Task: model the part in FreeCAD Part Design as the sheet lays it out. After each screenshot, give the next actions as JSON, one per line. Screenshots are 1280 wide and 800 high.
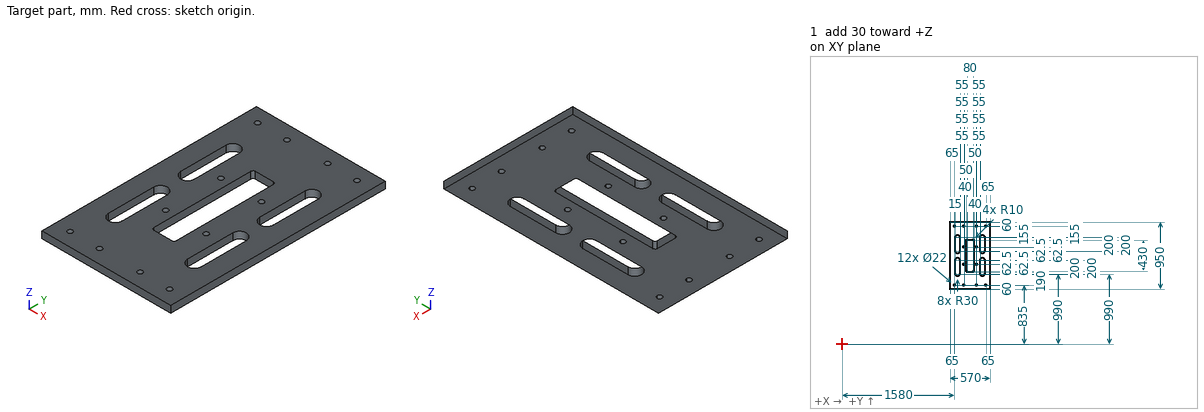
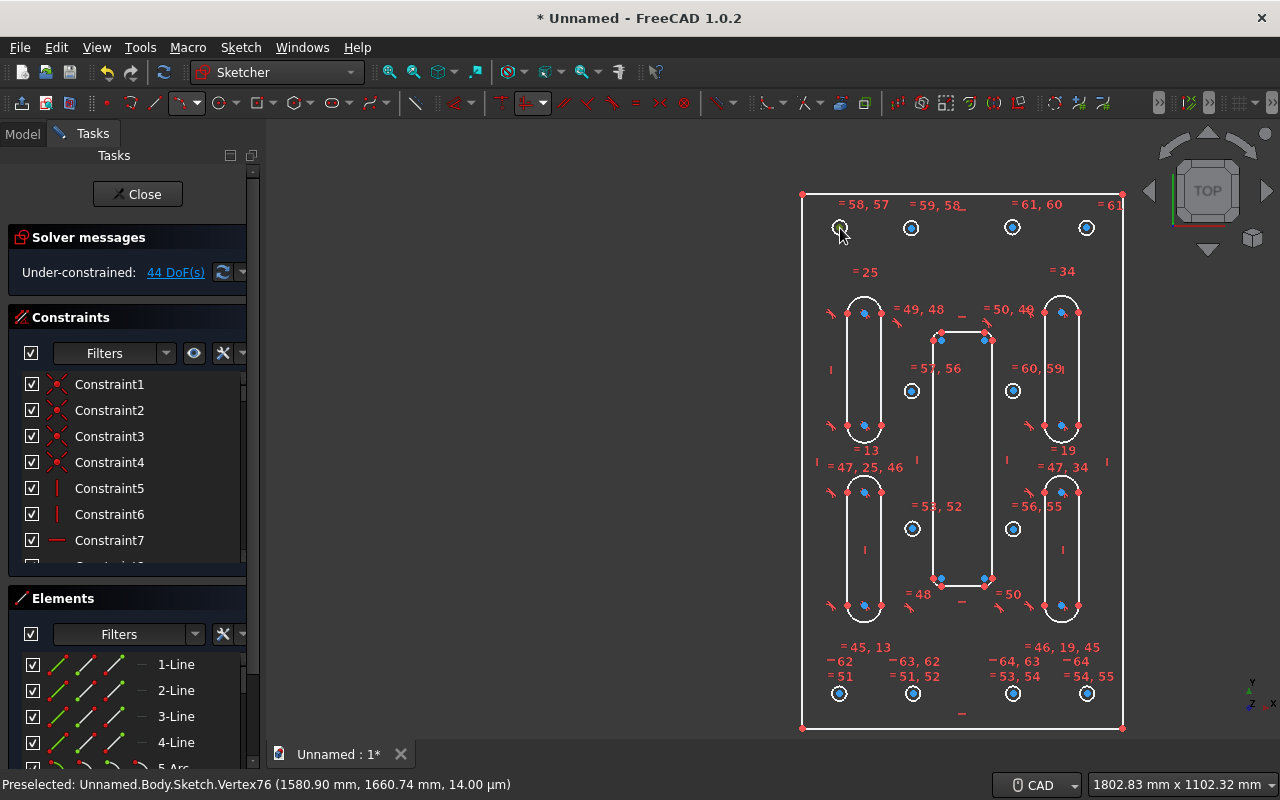
{"action": "left_click", "coordinate": [911, 228]}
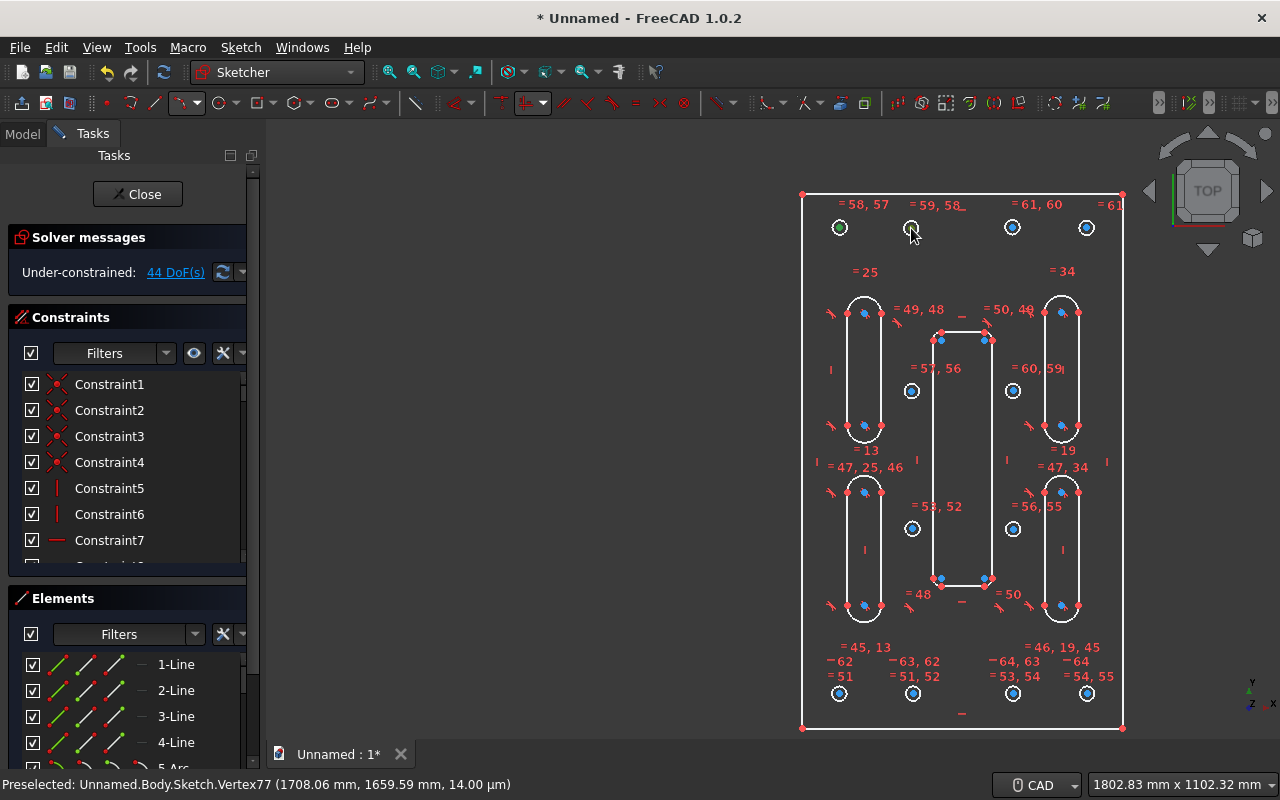
{"action": "key", "text": "h"}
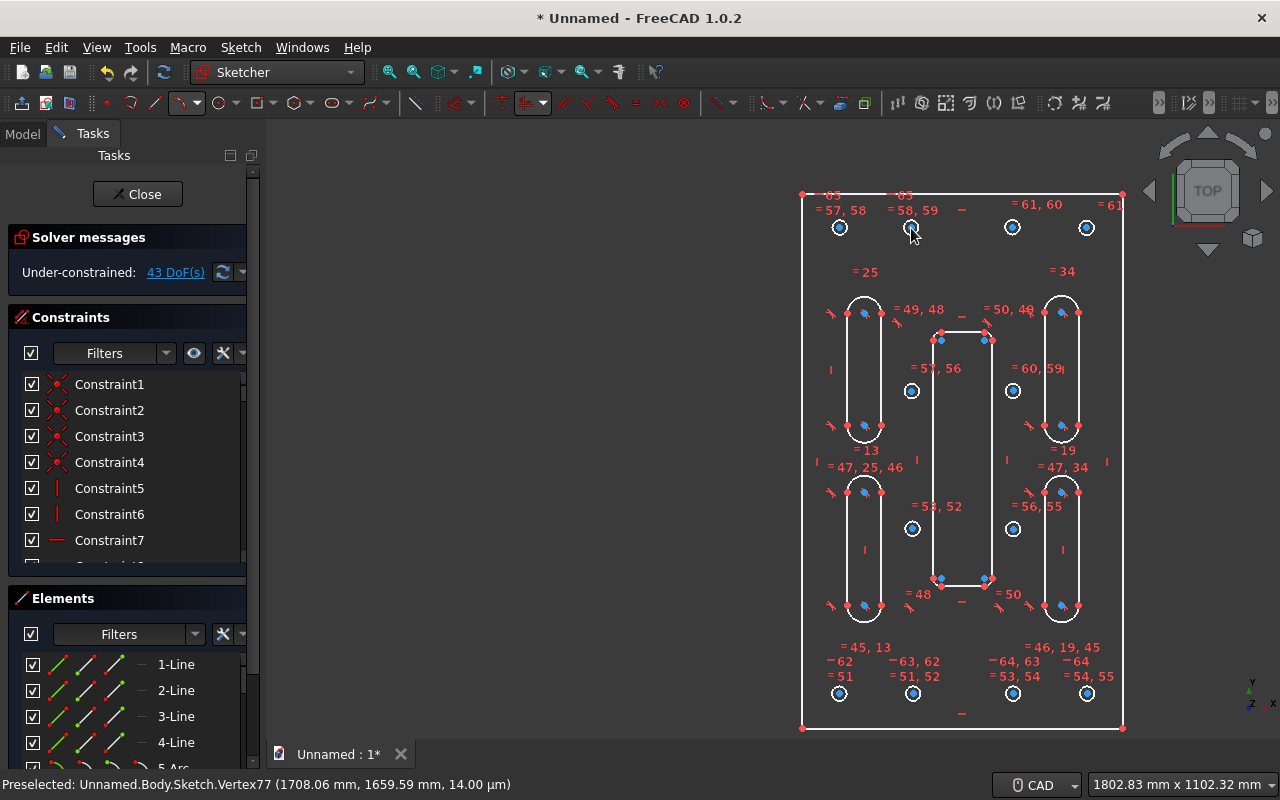
{"action": "left_click", "coordinate": [911, 228]}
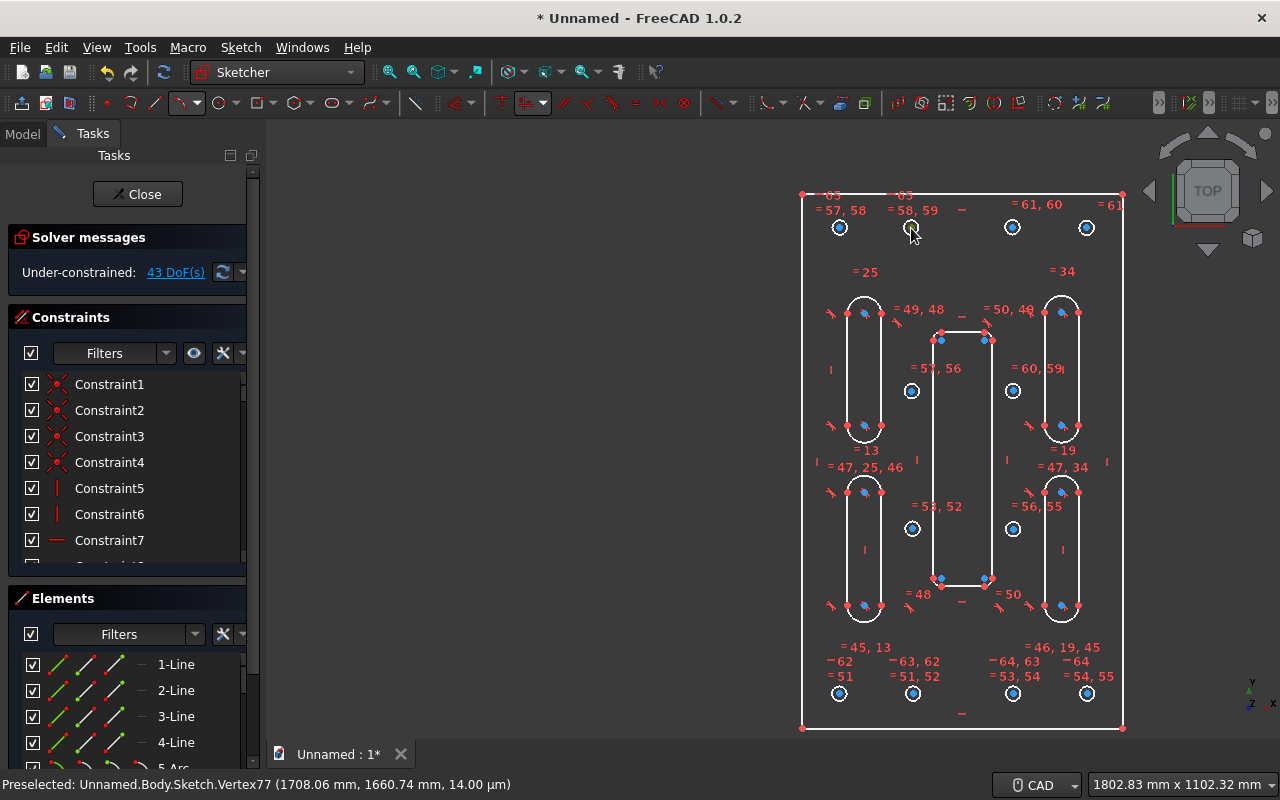
{"action": "left_click", "coordinate": [1012, 227]}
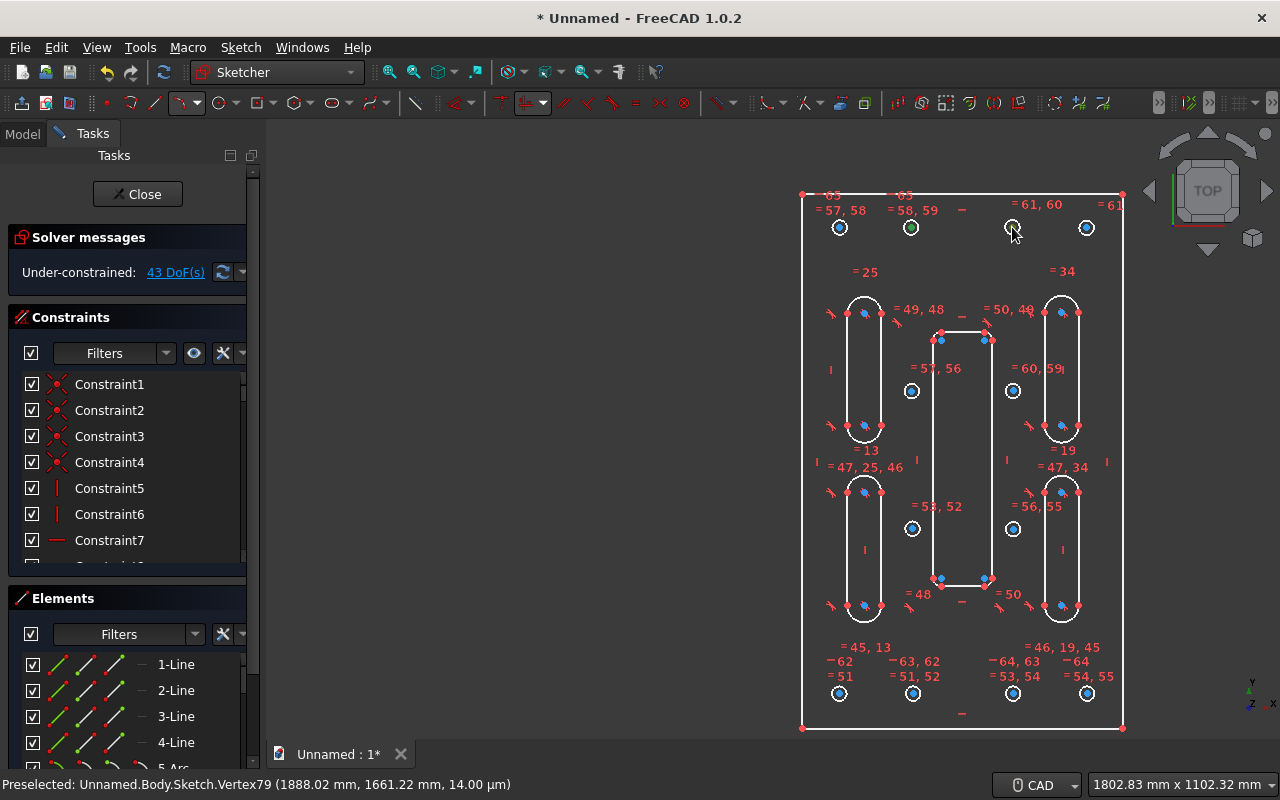
{"action": "key", "text": "h"}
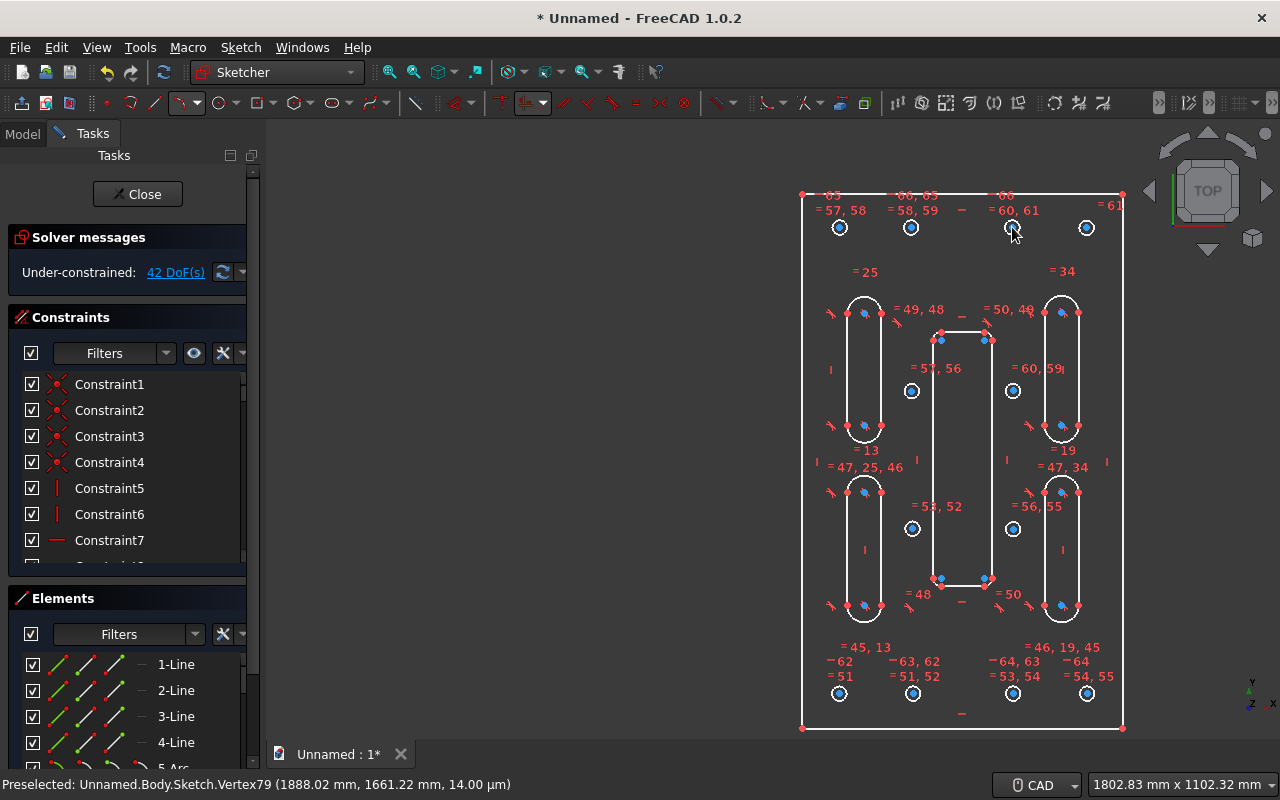
{"action": "left_click", "coordinate": [1012, 228]}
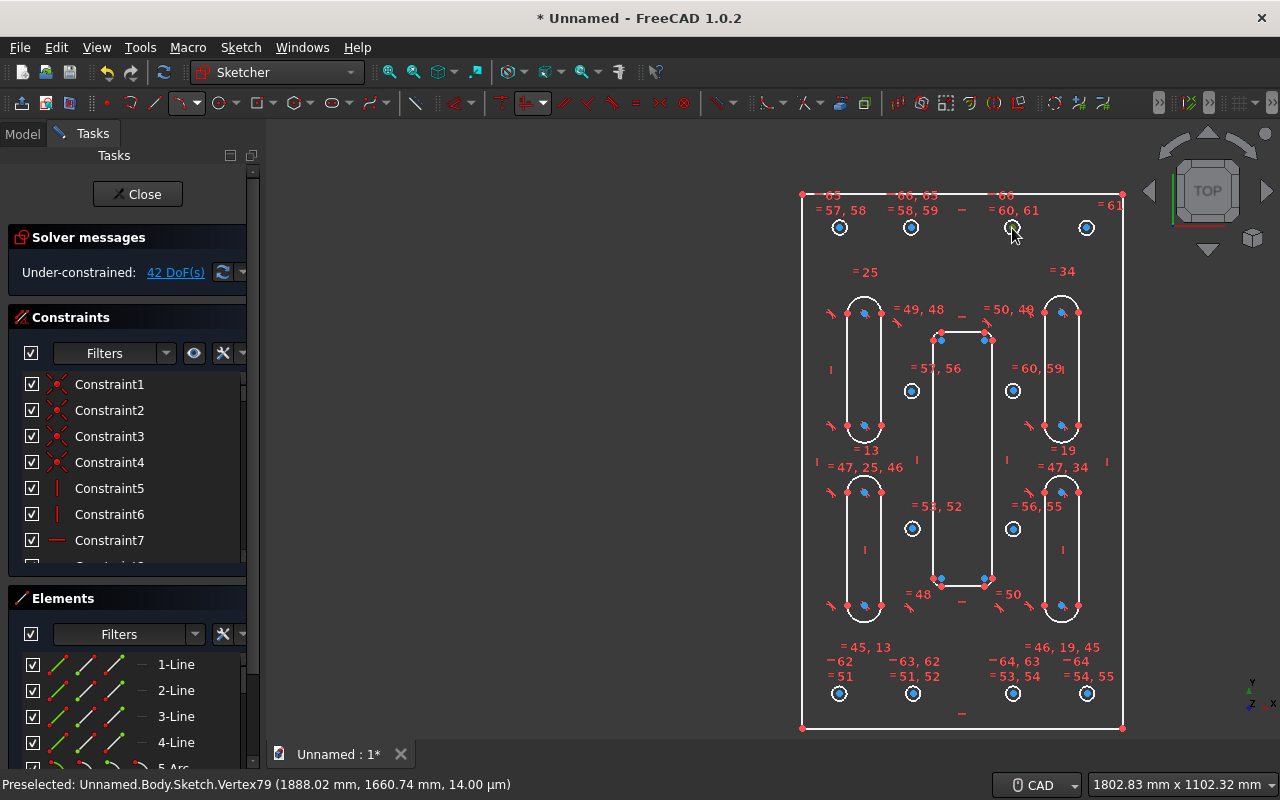
{"action": "left_click", "coordinate": [1087, 228]}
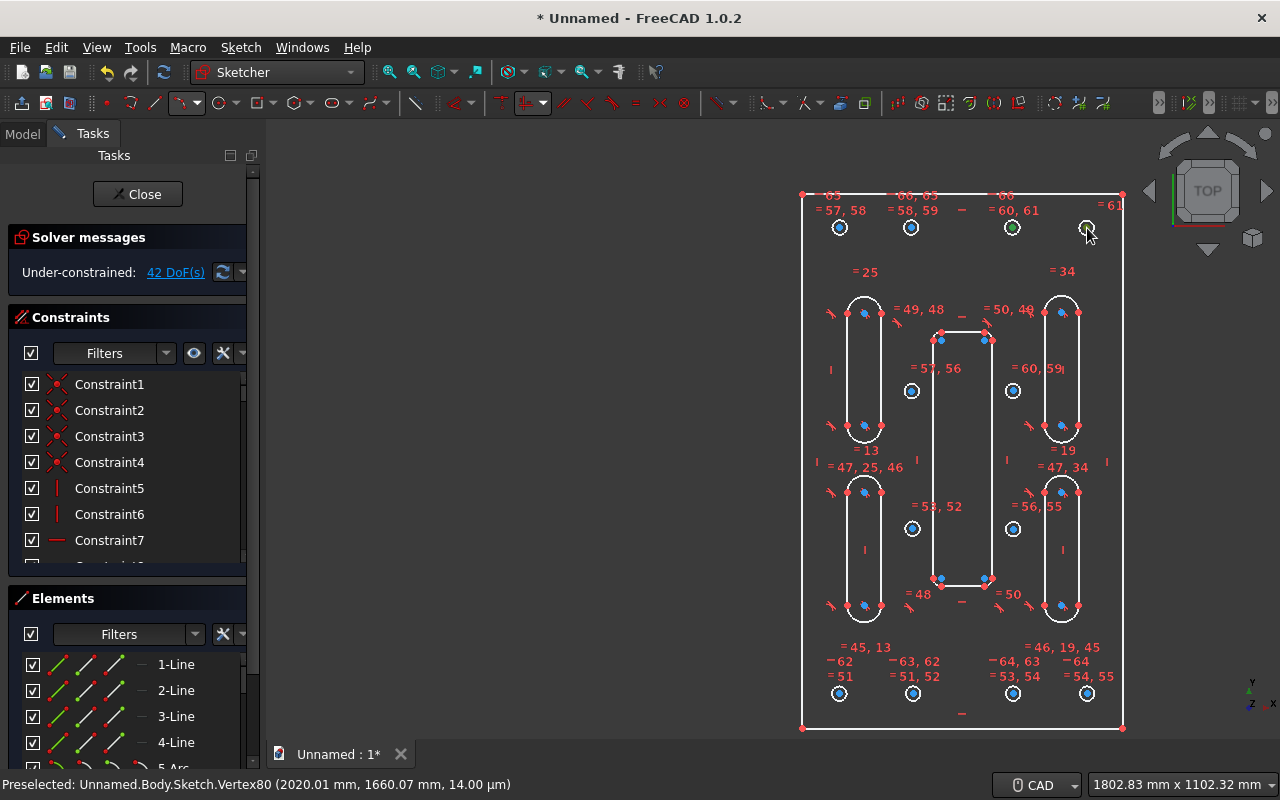
{"action": "key", "text": "h"}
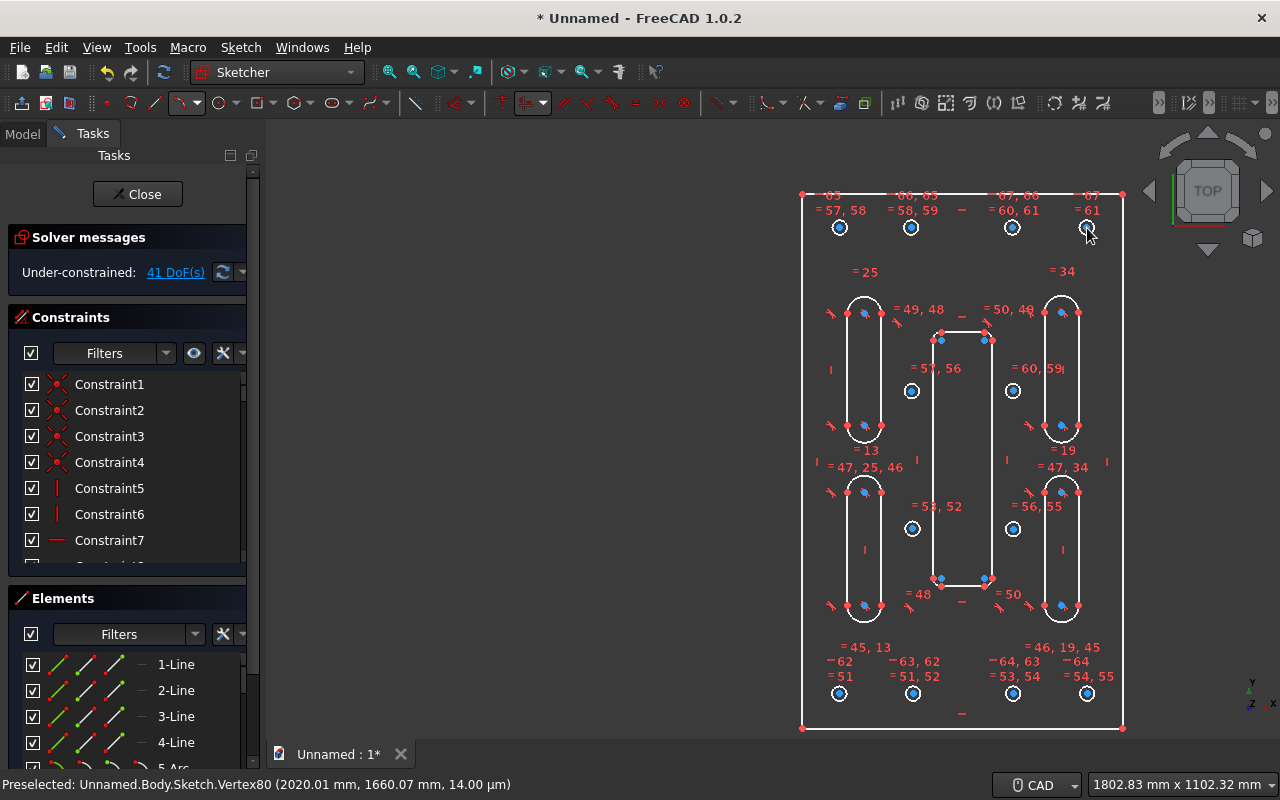
{"action": "key", "text": "d"}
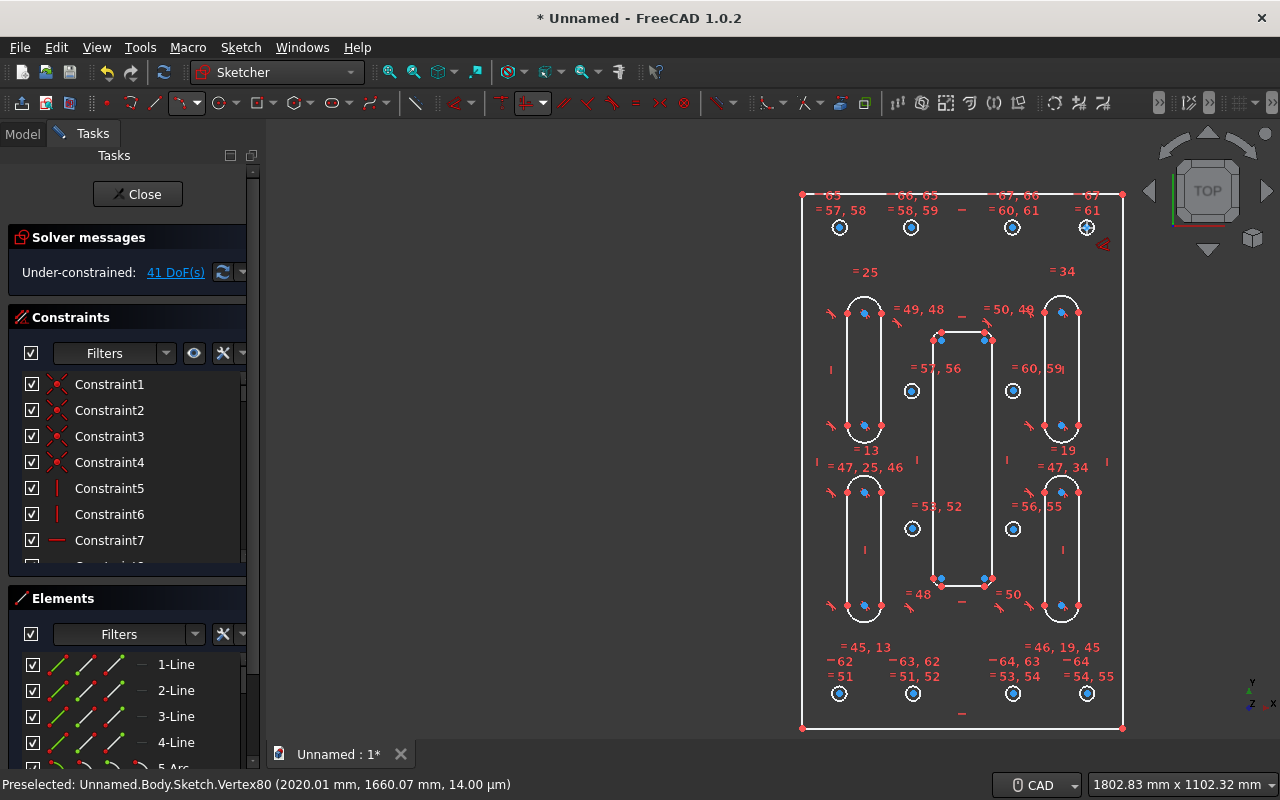
{"action": "scroll", "coordinate": [854, 619], "scroll_direction": "up", "scroll_amount": 5}